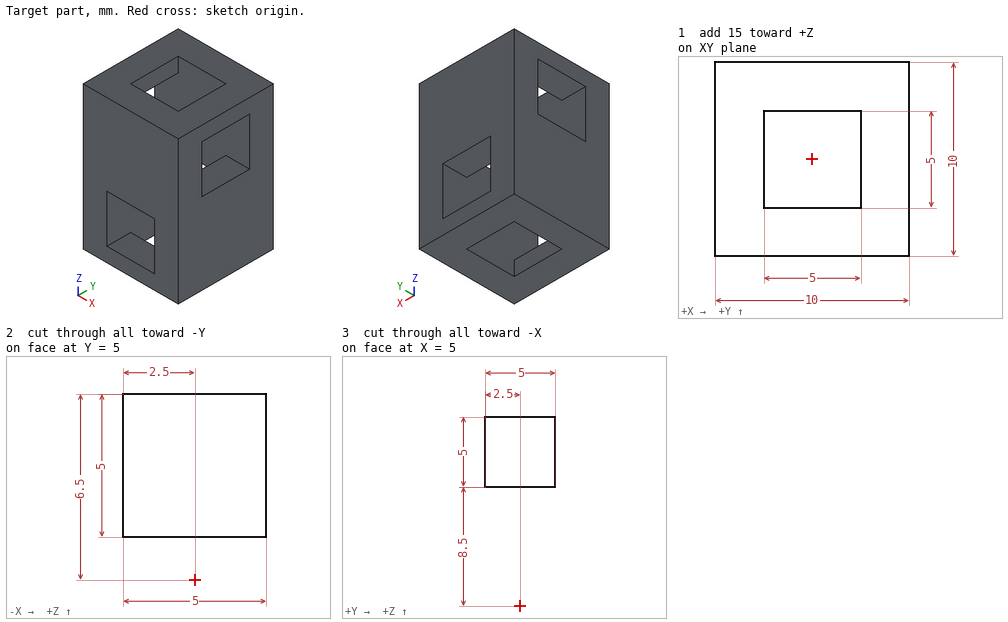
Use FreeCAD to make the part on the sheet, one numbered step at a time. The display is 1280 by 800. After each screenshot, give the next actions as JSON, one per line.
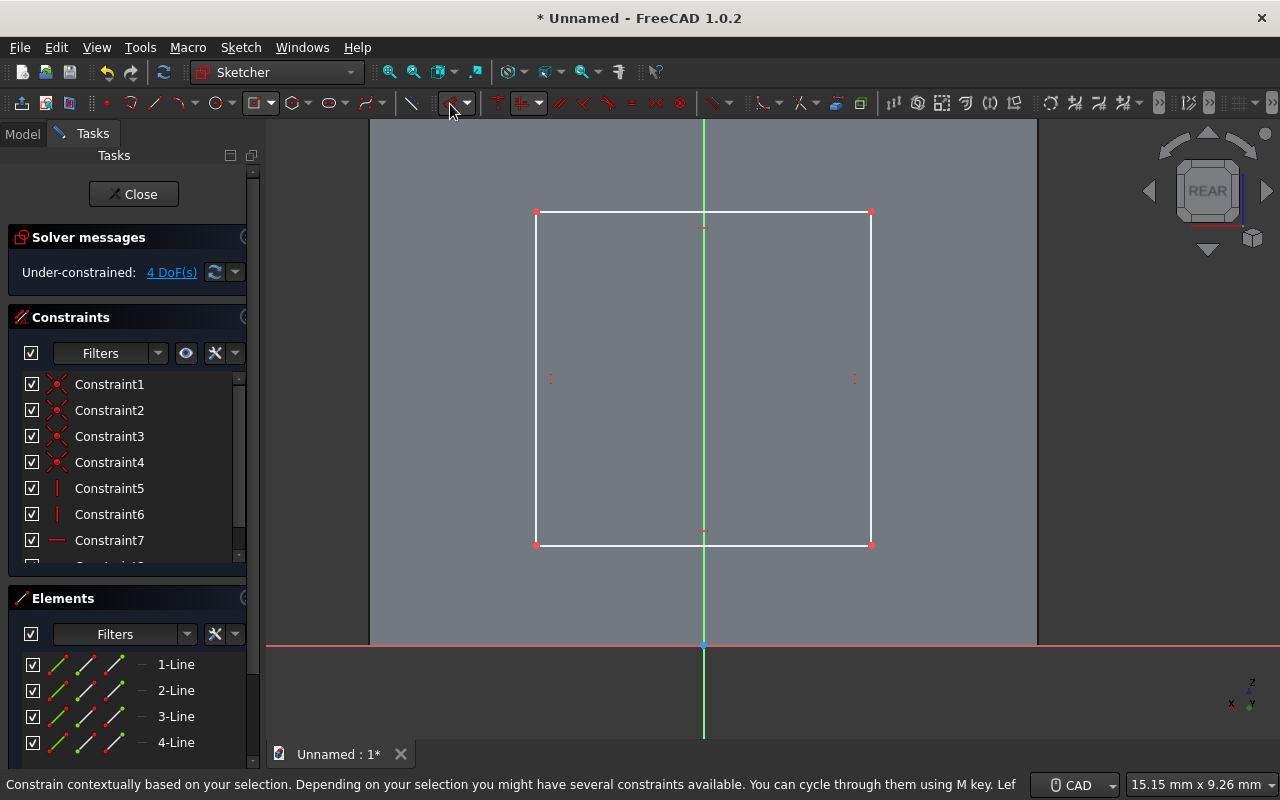
{"action": "left_click", "coordinate": [536, 312]}
{"action": "left_click", "coordinate": [502, 379]}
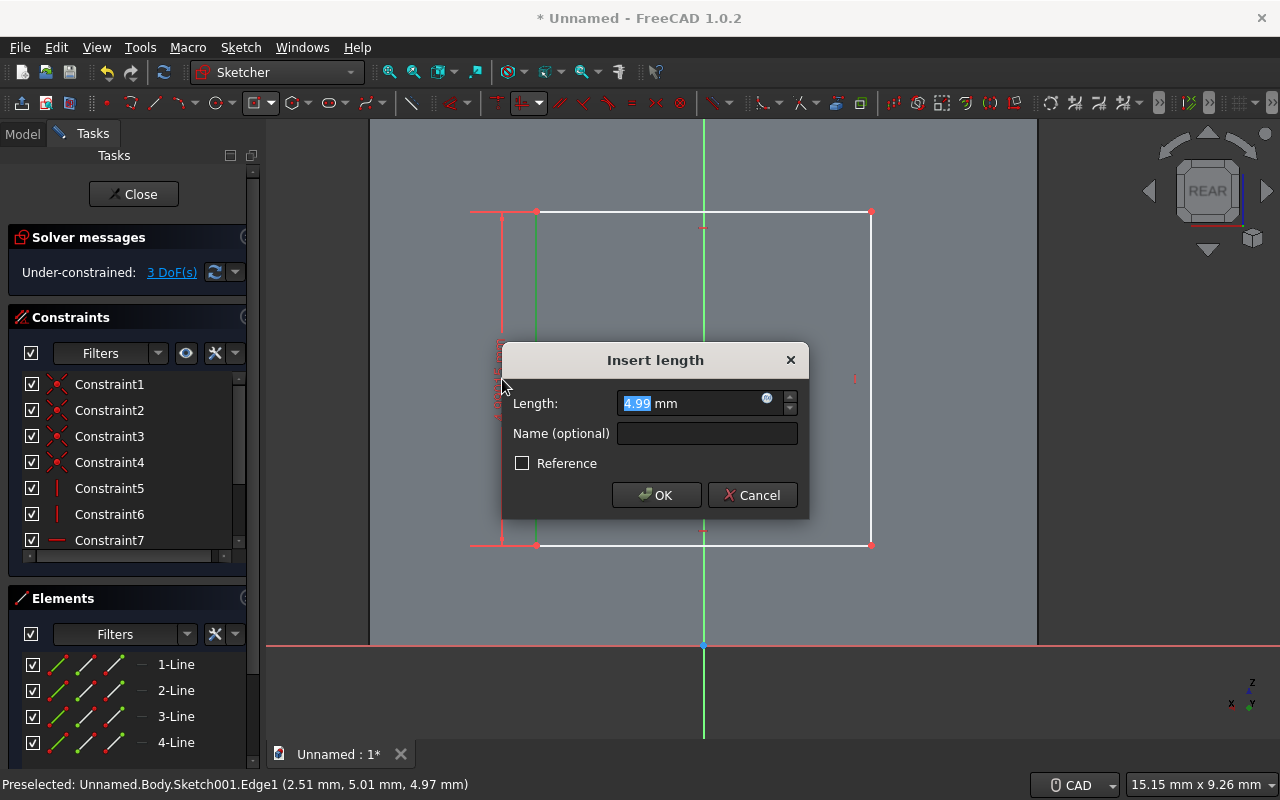
{"action": "type", "text": "5"}
{"action": "key", "text": "Return"}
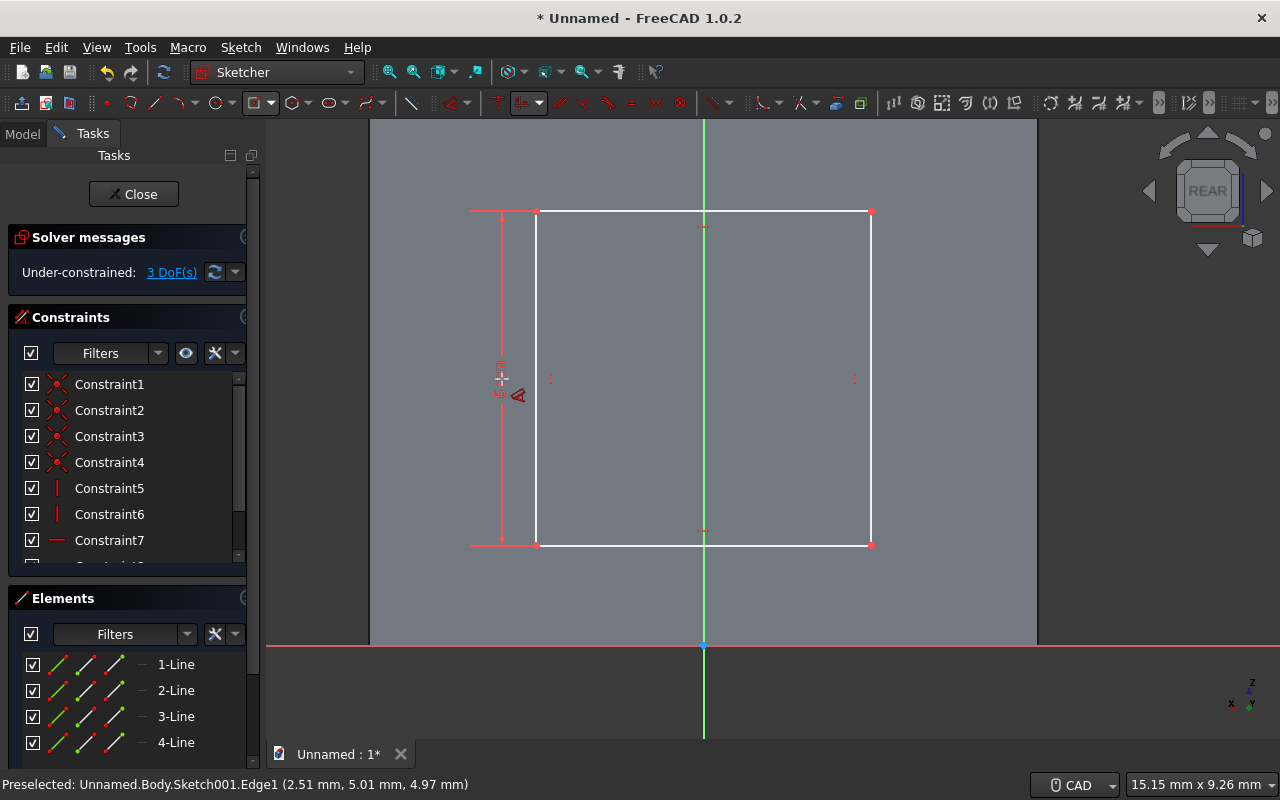
{"action": "left_click", "coordinate": [637, 546]}
{"action": "left_click", "coordinate": [626, 580]}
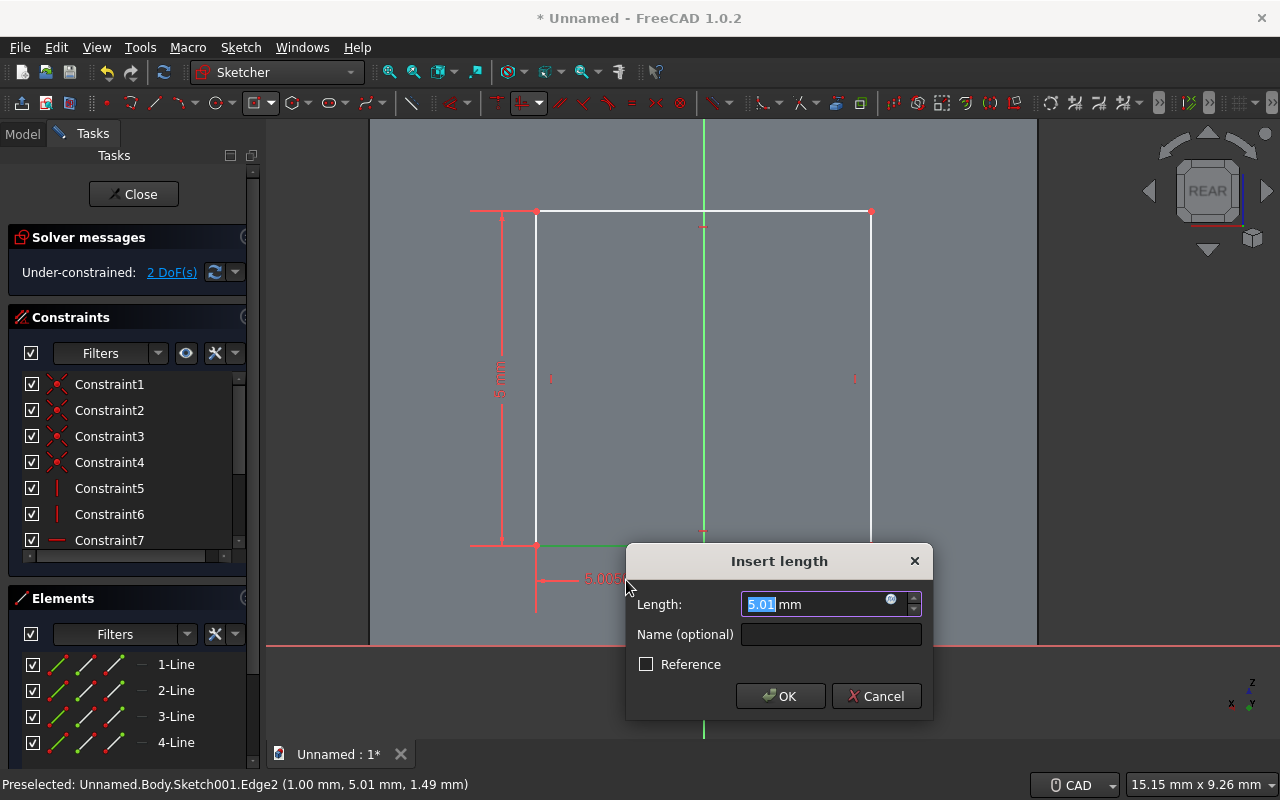
{"action": "type", "text": "5"}
{"action": "key", "text": "Return"}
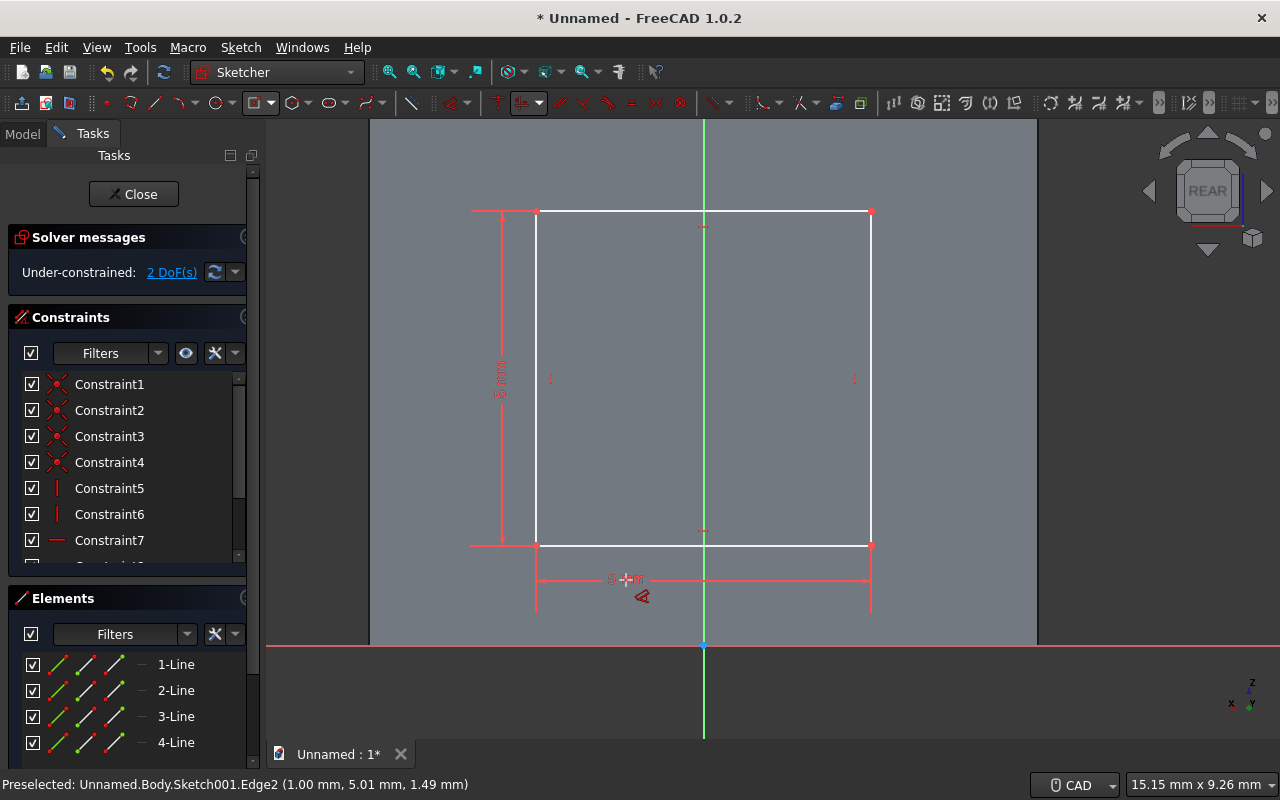
{"action": "left_click", "coordinate": [536, 211]}
{"action": "left_click", "coordinate": [620, 680]}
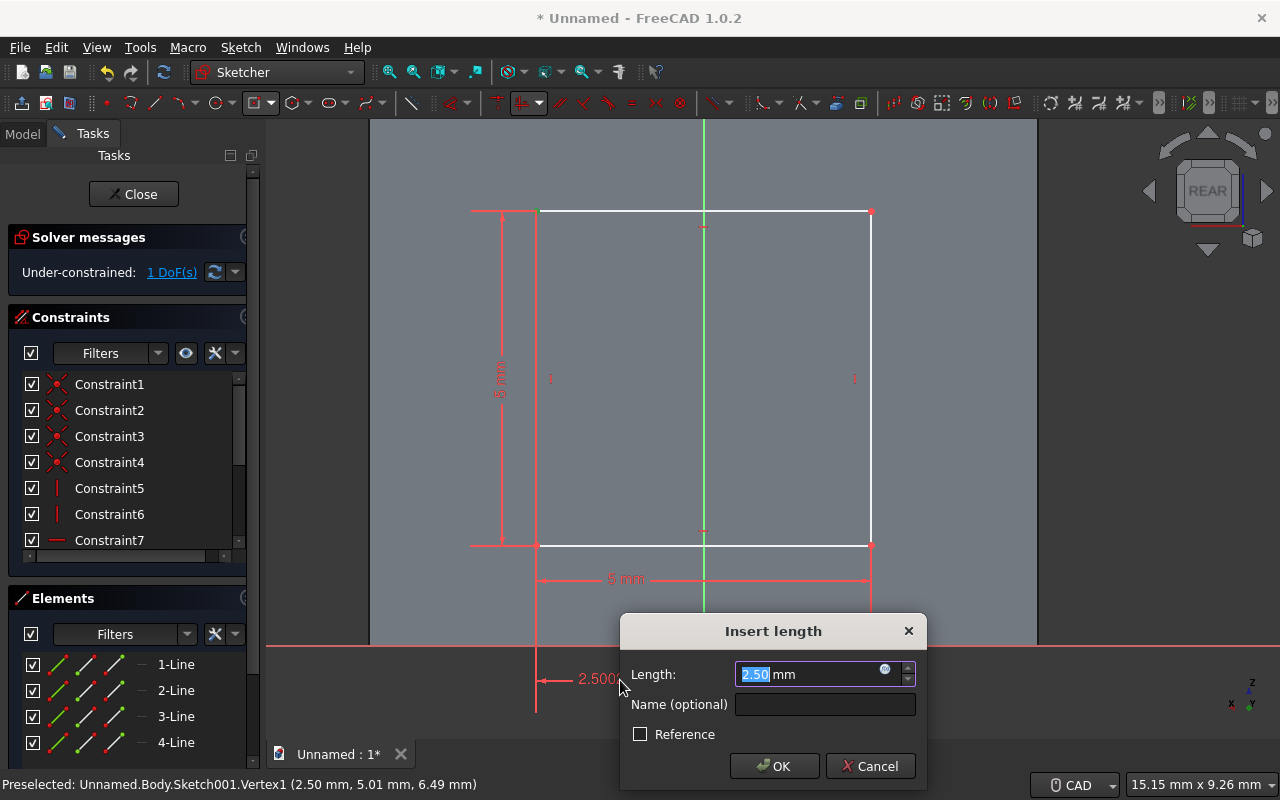
{"action": "type", "text": "2.5"}
{"action": "key", "text": "Return"}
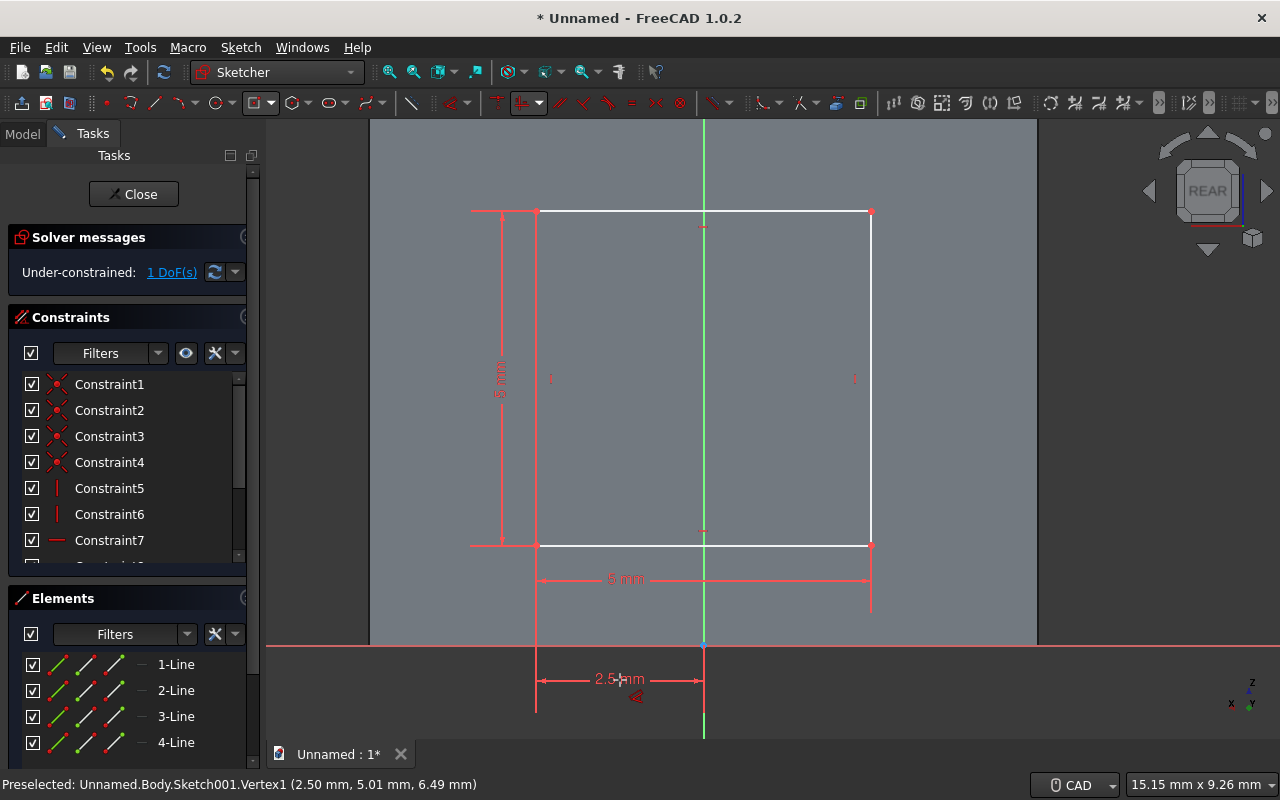
{"action": "left_click", "coordinate": [536, 211]}
{"action": "left_click", "coordinate": [502, 428]}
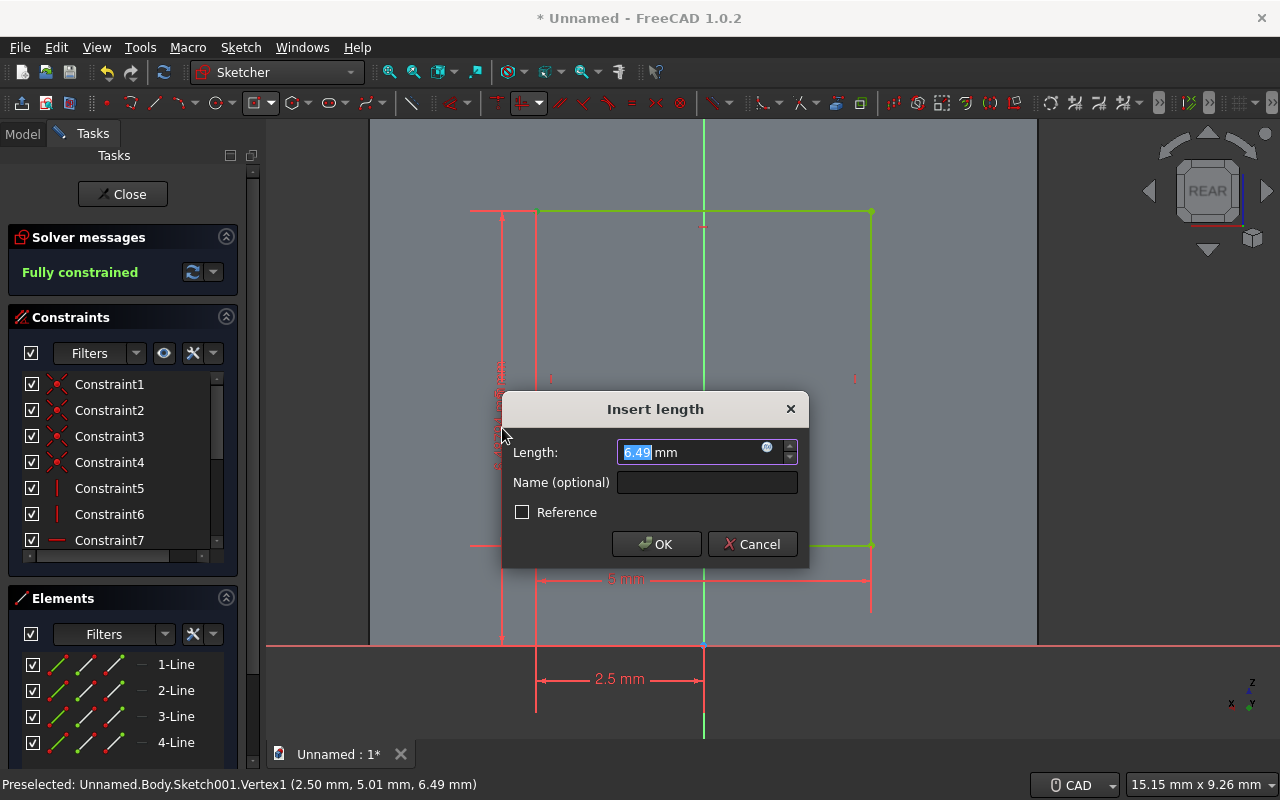
{"action": "type", "text": "6.5"}
{"action": "key", "text": "Return"}
{"action": "key", "text": "Escape"}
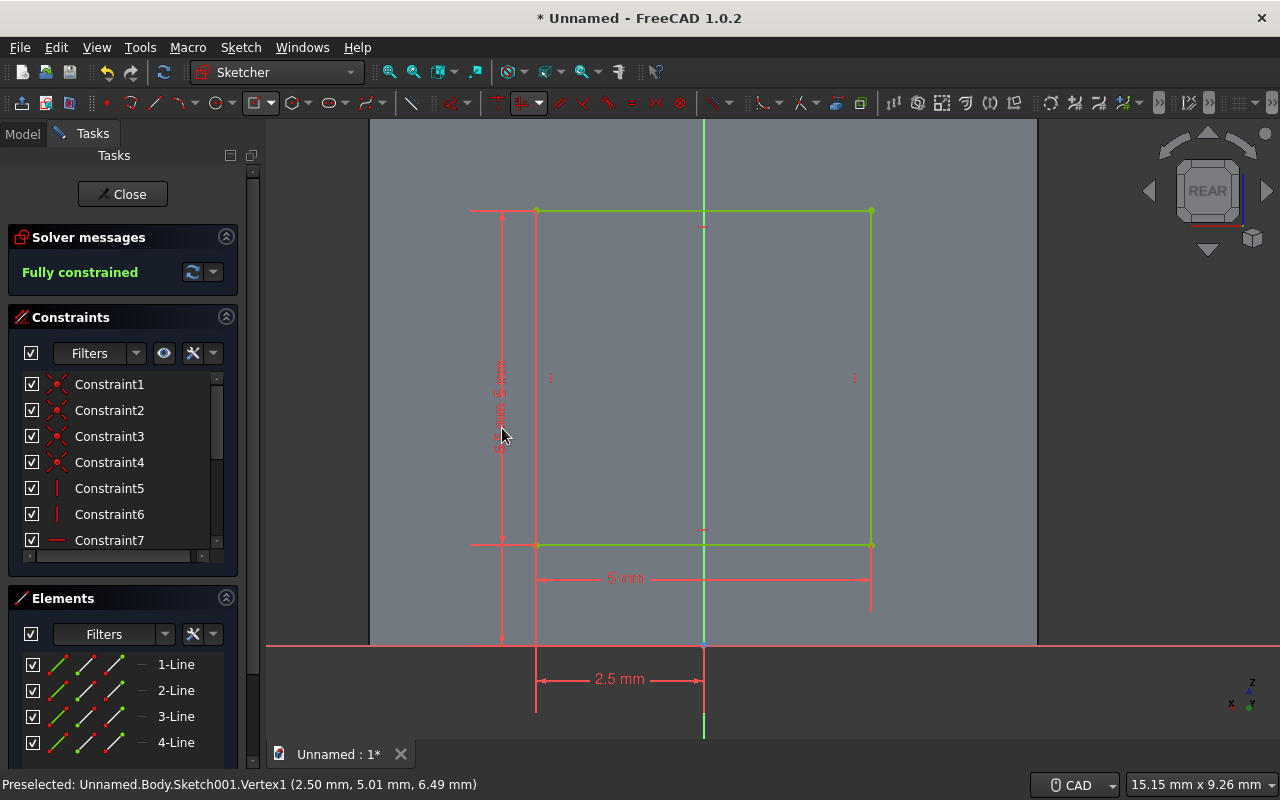
{"action": "left_click", "coordinate": [123, 194]}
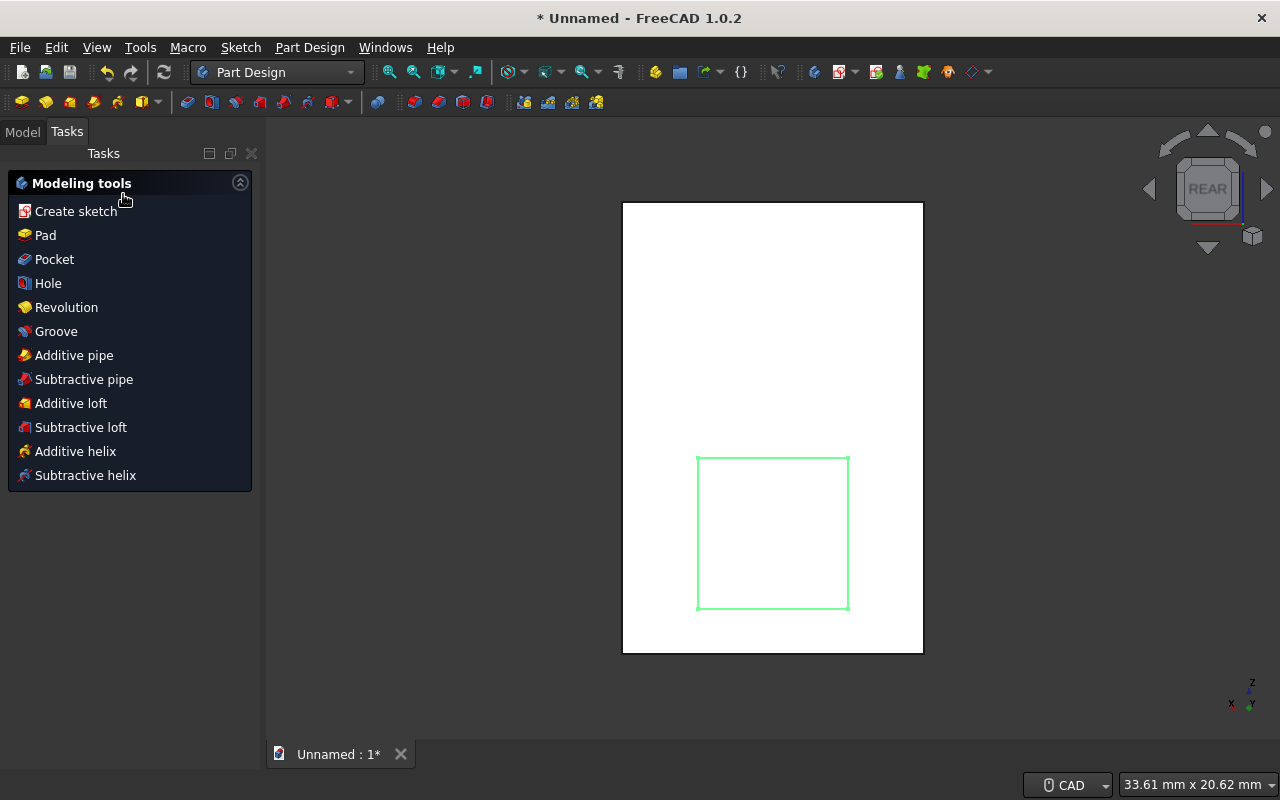
{"action": "left_click", "coordinate": [188, 102]}